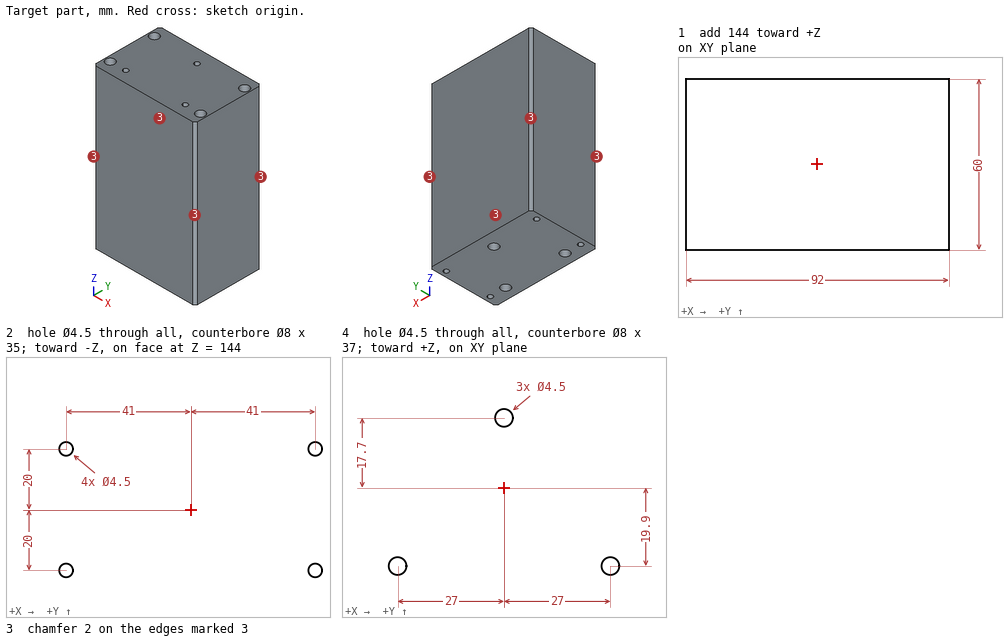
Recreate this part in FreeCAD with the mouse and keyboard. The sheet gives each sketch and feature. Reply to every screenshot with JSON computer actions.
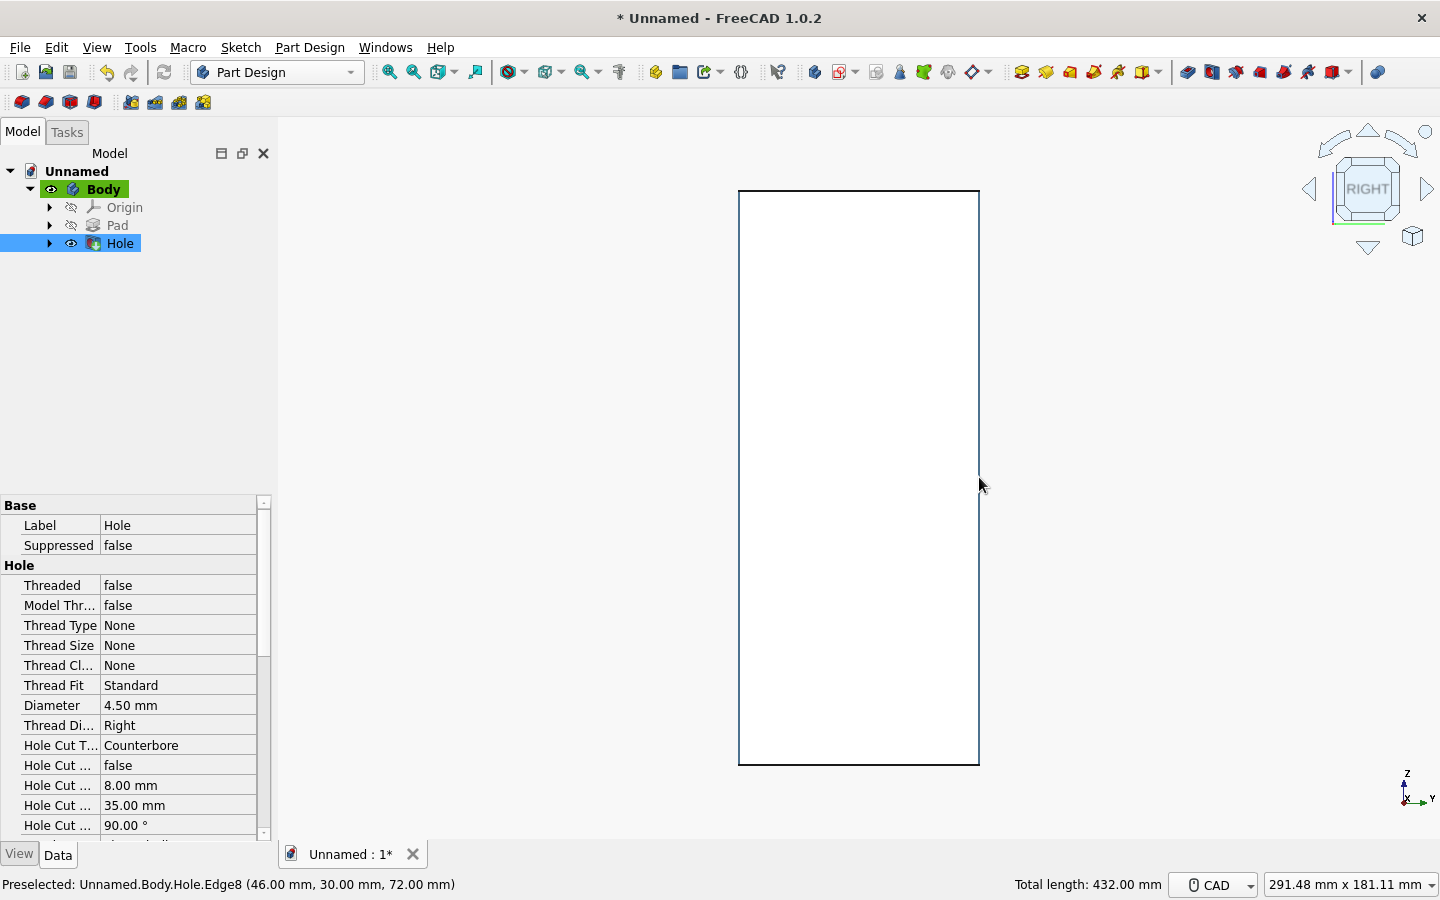
{"action": "key", "text": "5"}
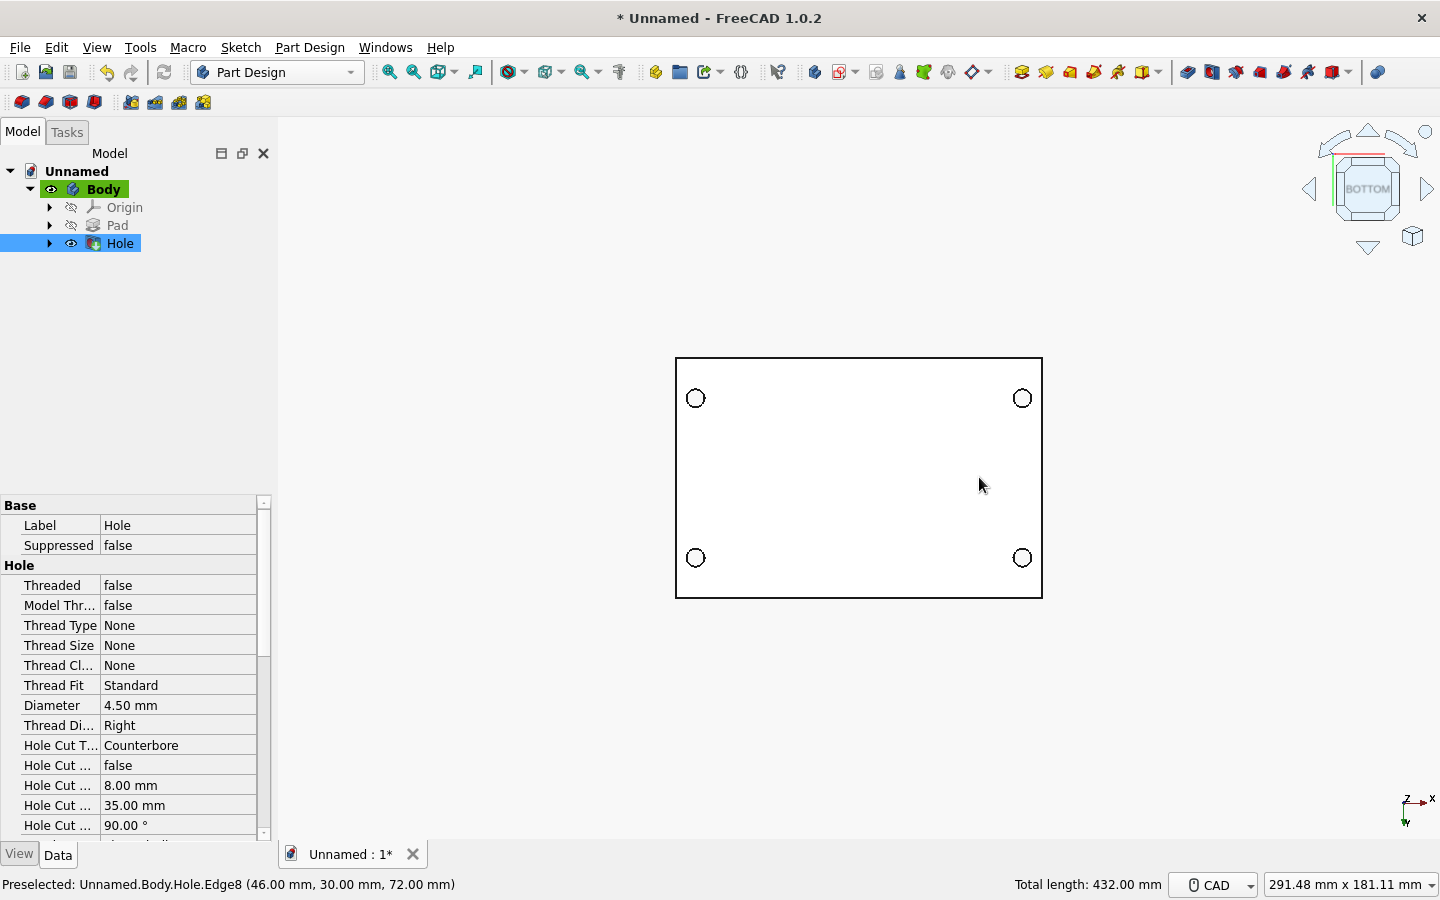
{"action": "left_click", "coordinate": [390, 72]}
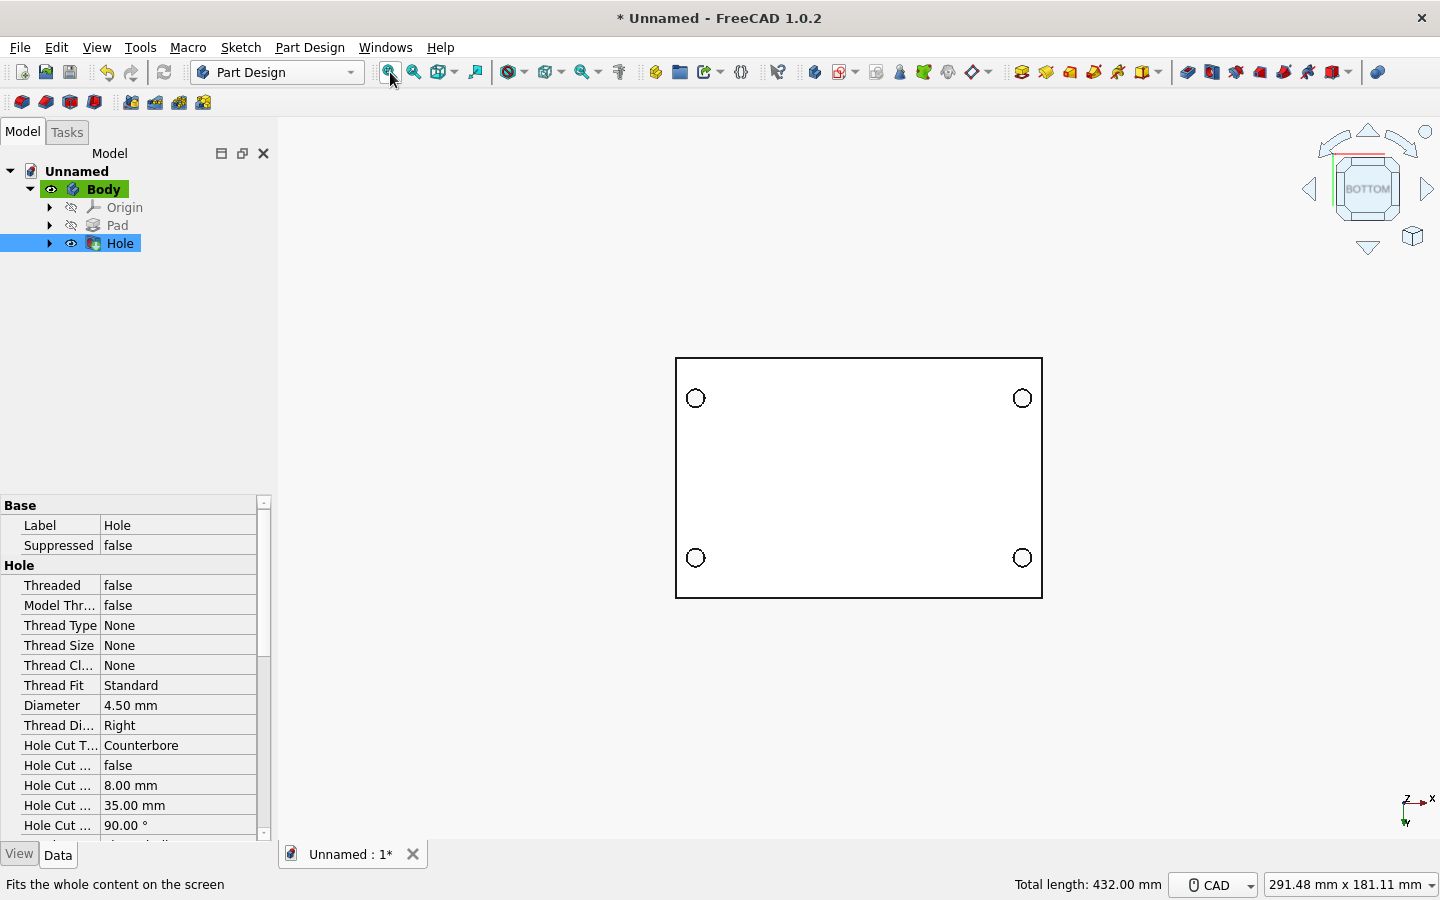
{"action": "key", "text": "4"}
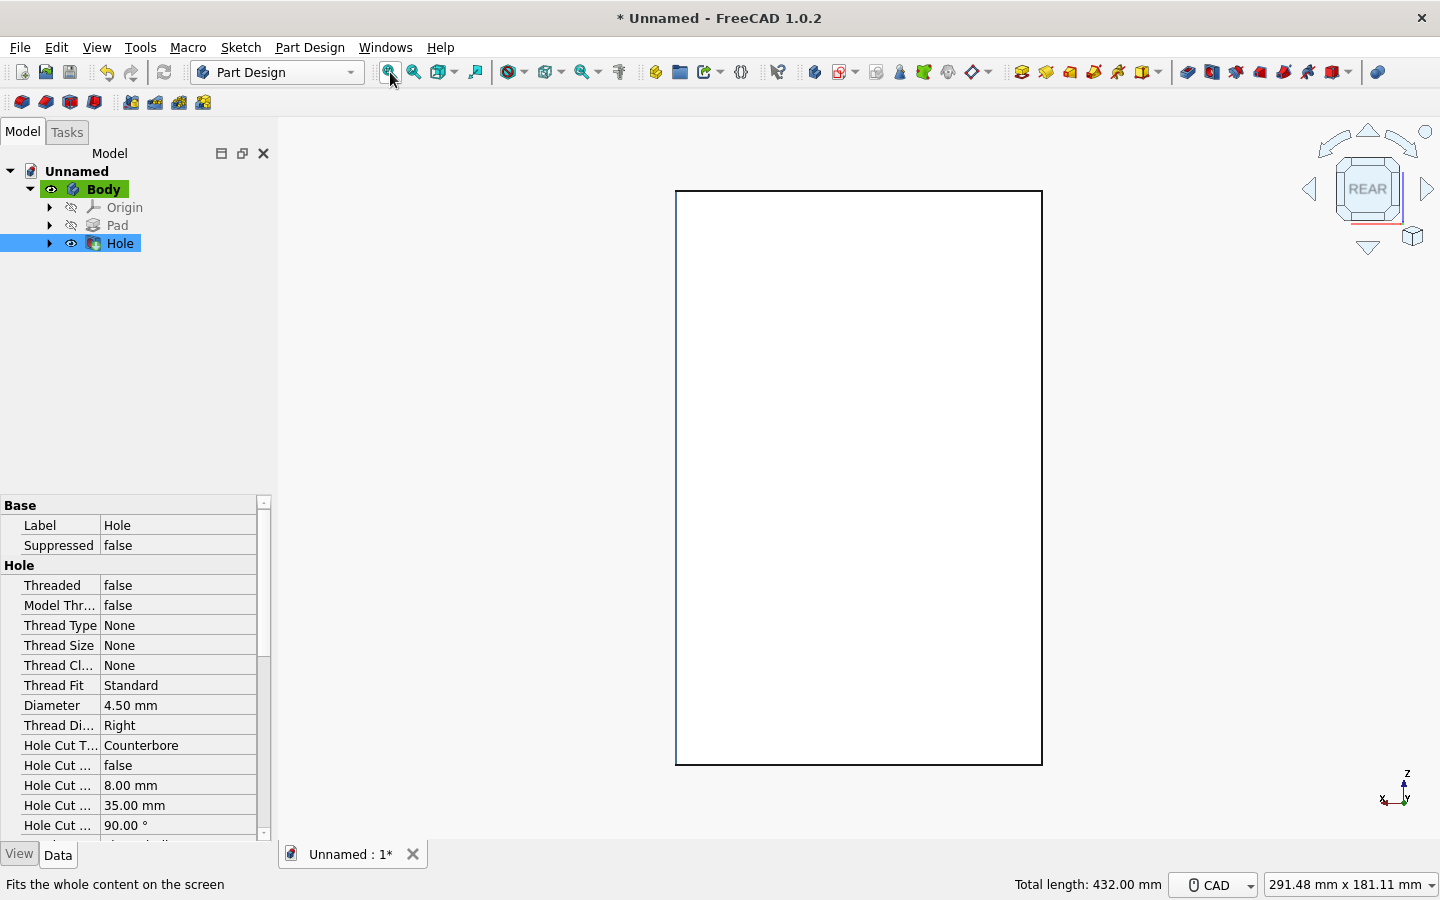
{"action": "left_click", "coordinate": [1042, 477], "text": "ctrl"}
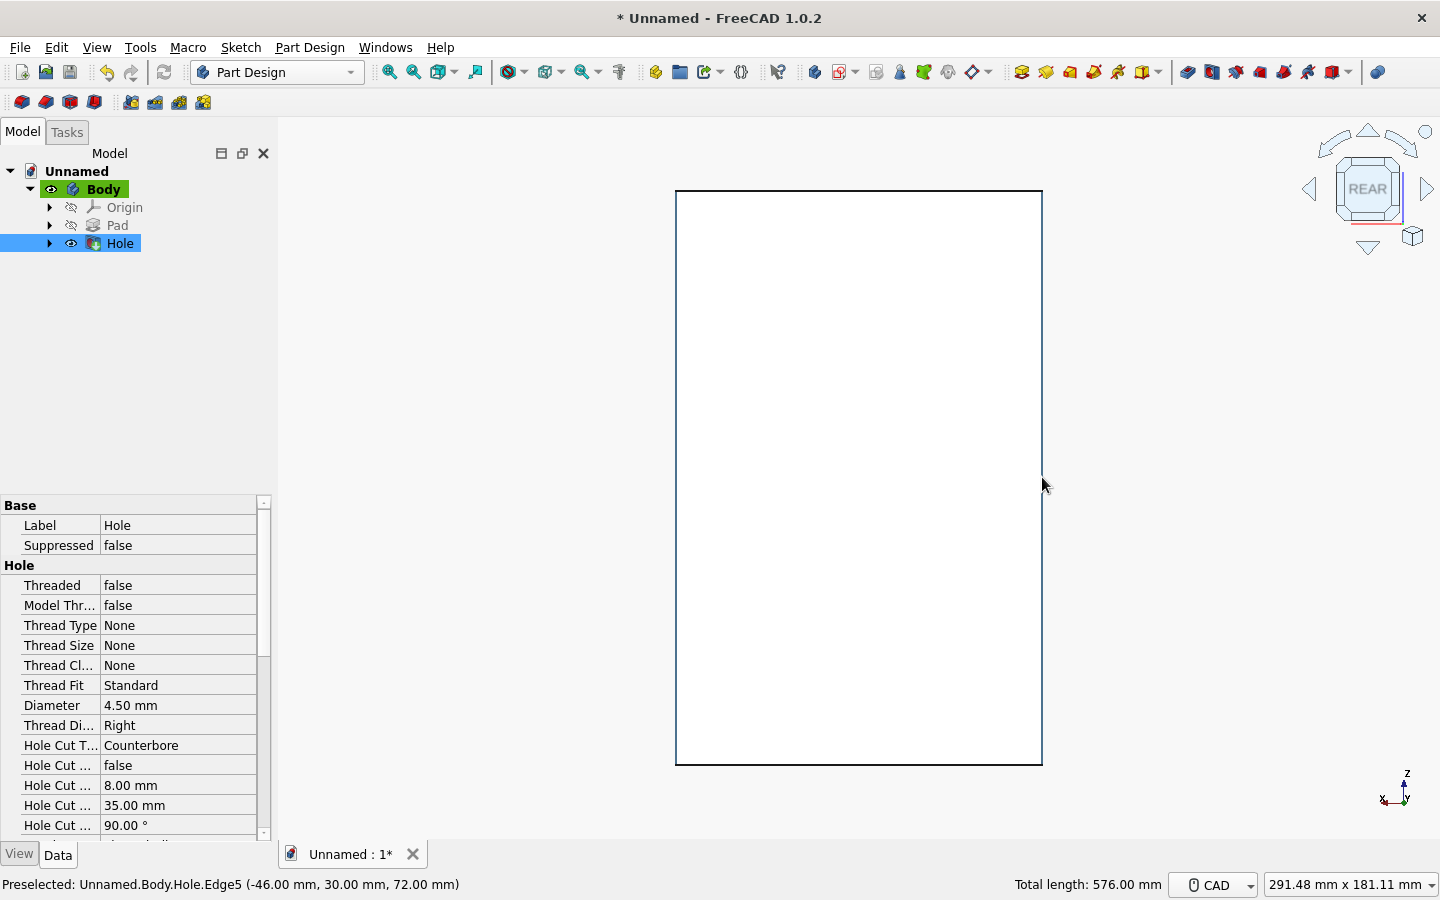
{"action": "left_click", "coordinate": [46, 102]}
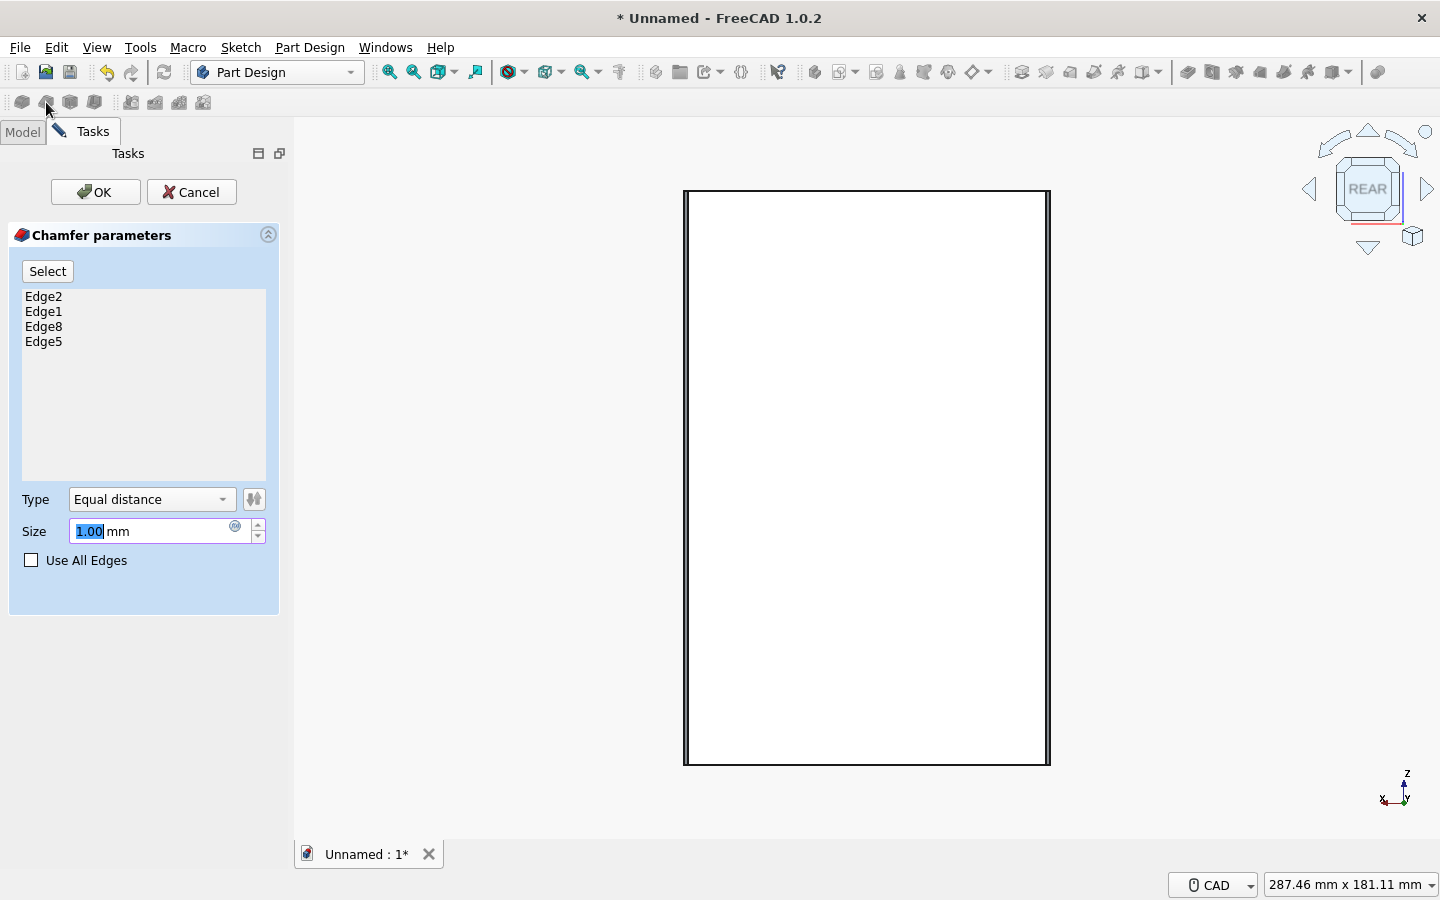
{"action": "type", "text": "2"}
{"action": "key", "text": "Tab"}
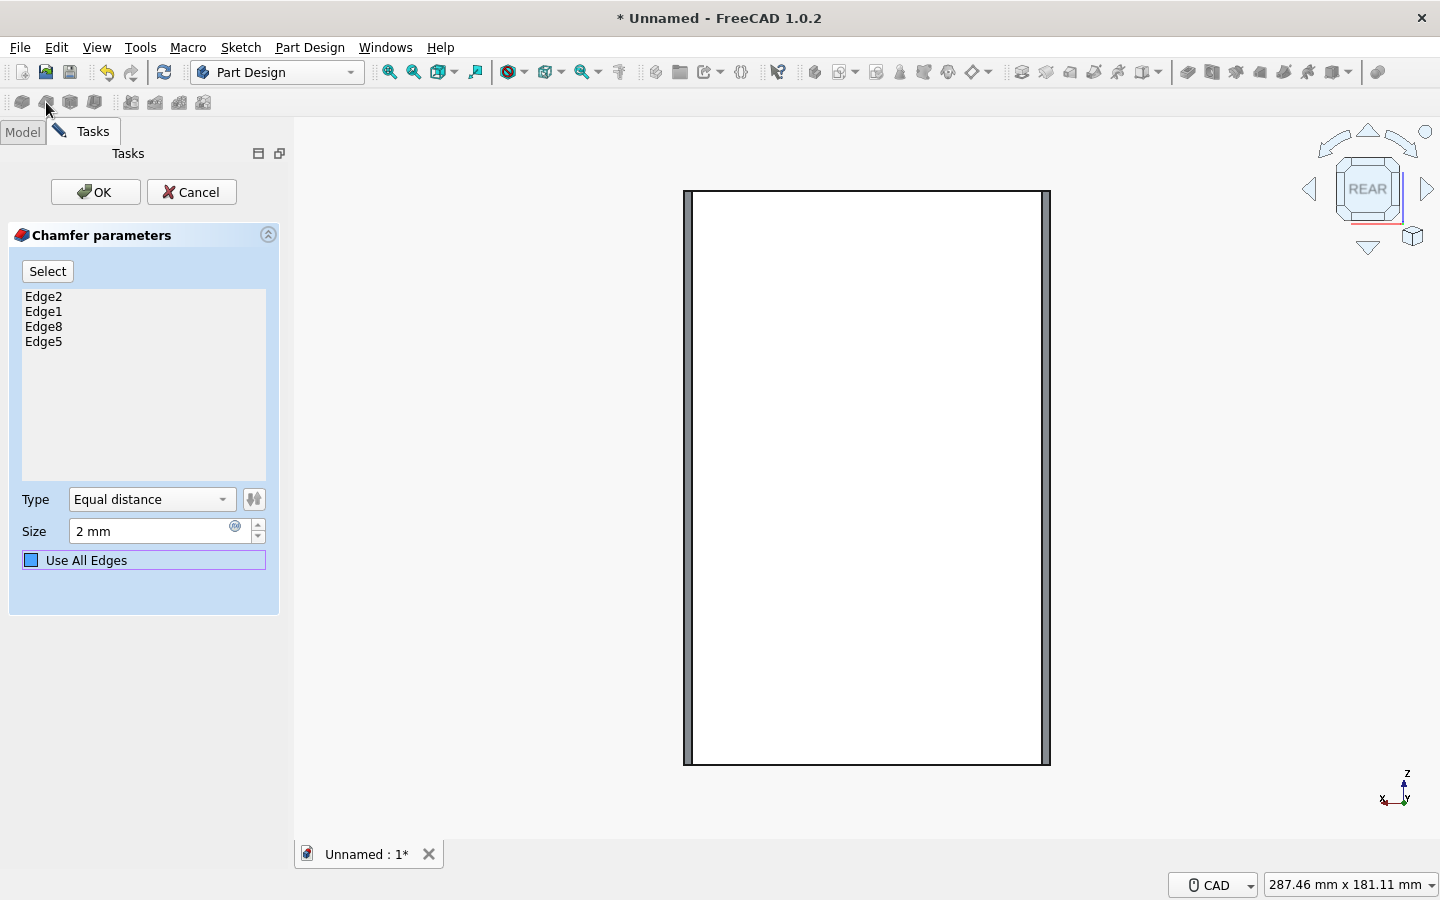
{"action": "left_click", "coordinate": [96, 192]}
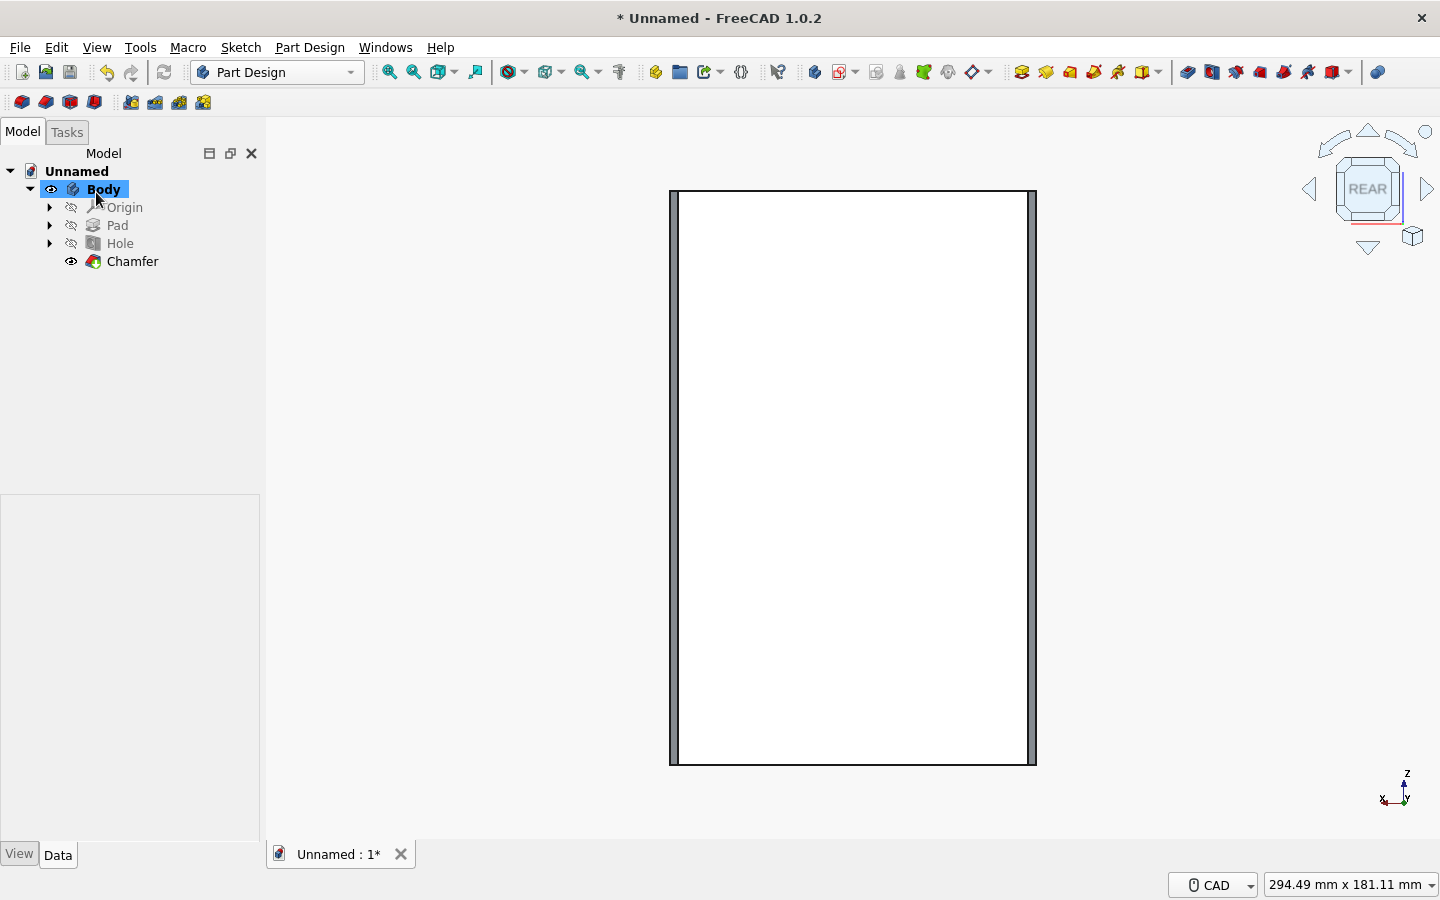
{"action": "left_click", "coordinate": [840, 72]}